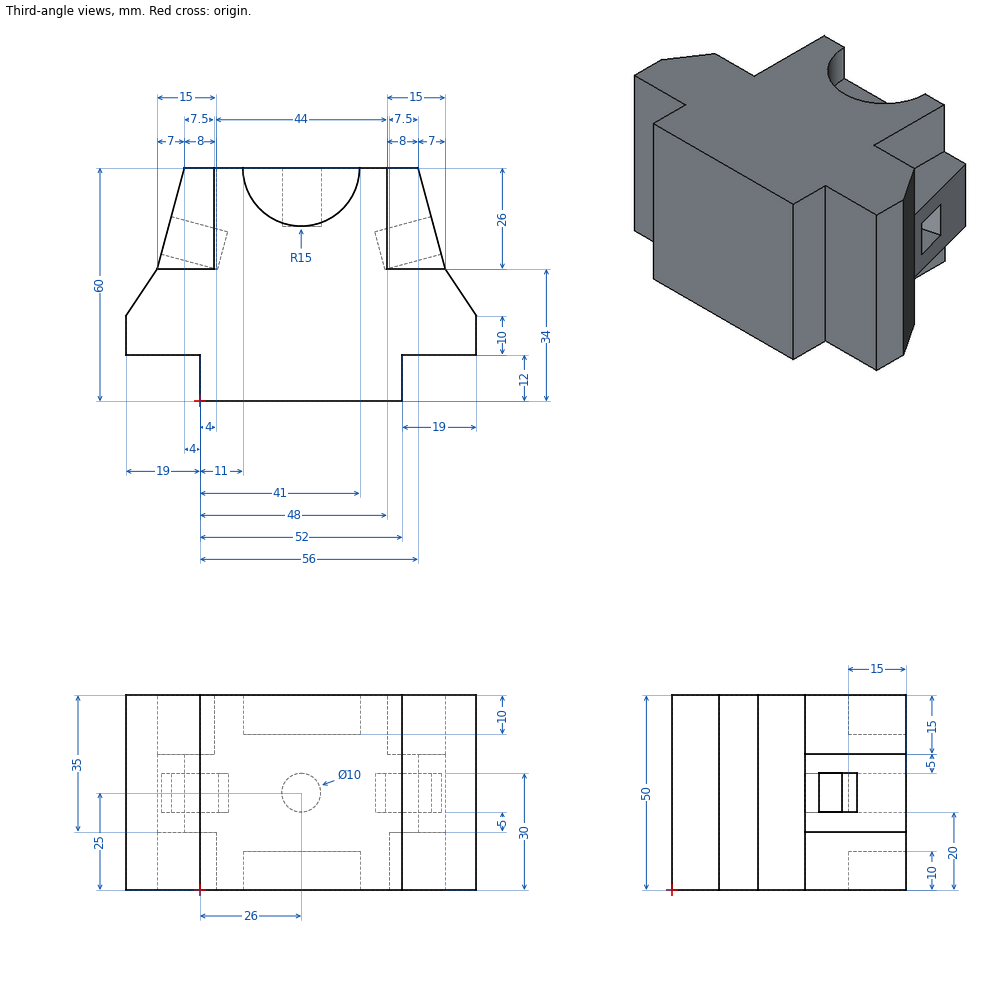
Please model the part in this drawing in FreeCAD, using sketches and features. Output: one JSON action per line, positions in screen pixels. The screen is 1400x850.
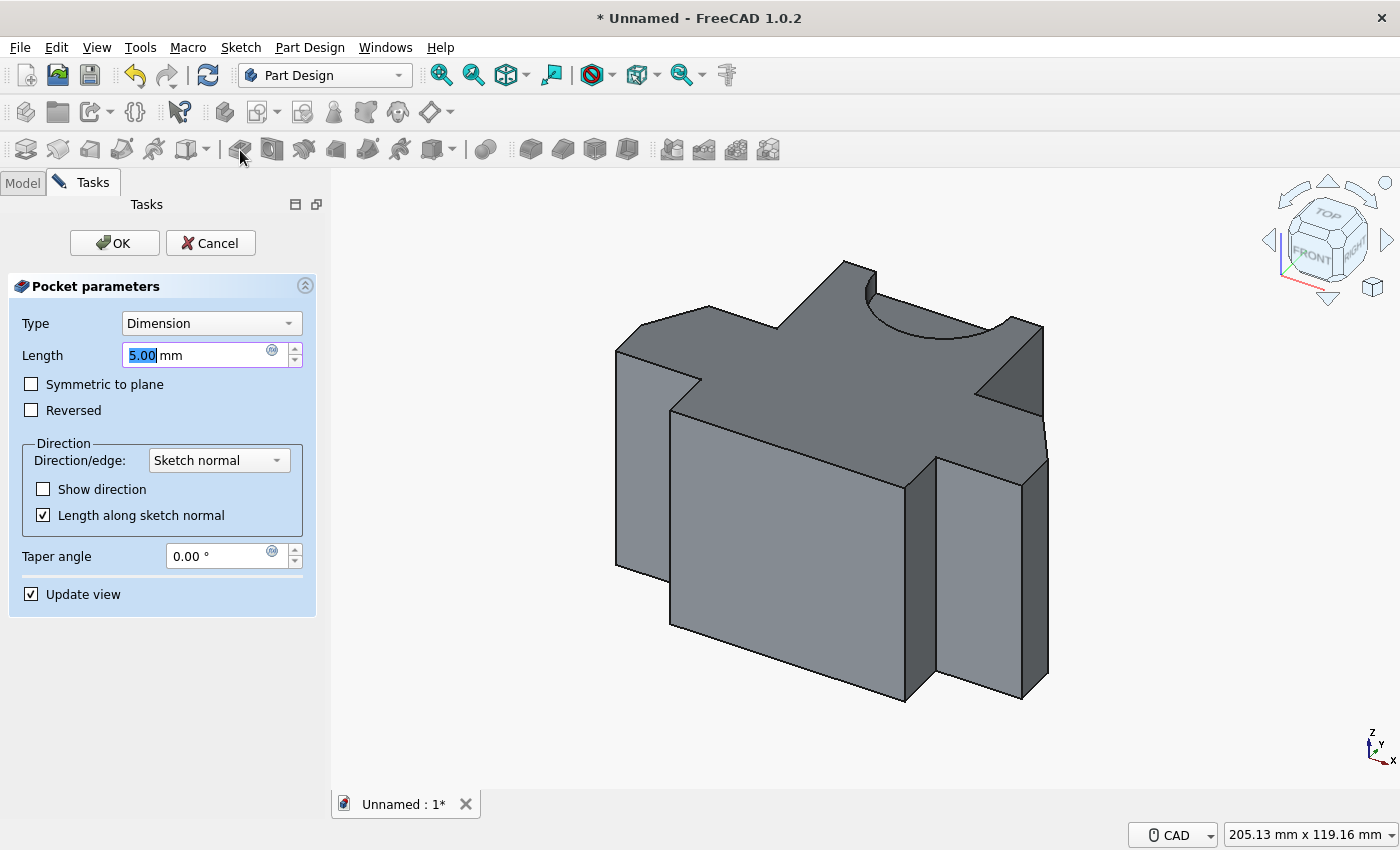
{"action": "type", "text": "10"}
{"action": "key", "text": "Tab"}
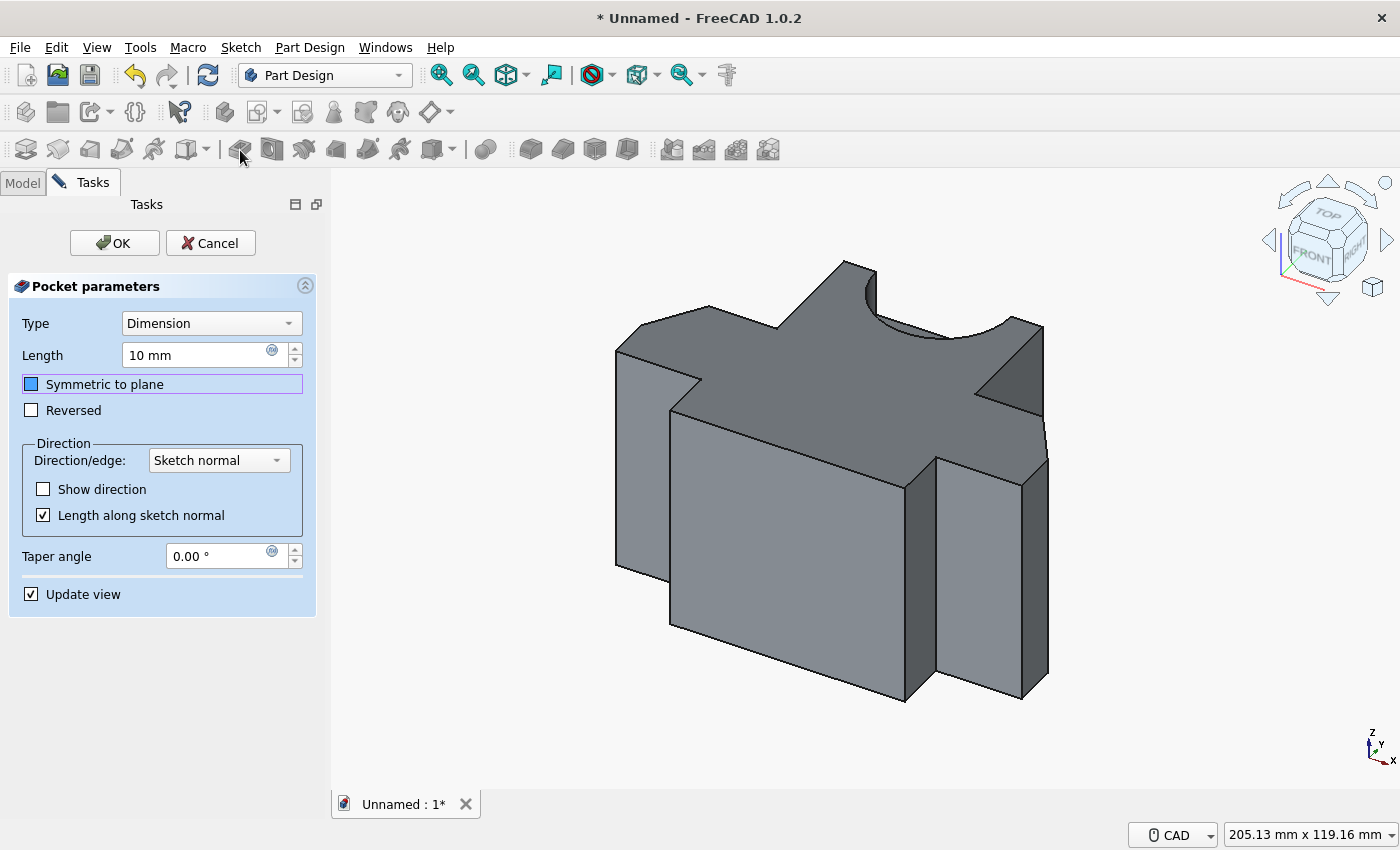
{"action": "left_click", "coordinate": [115, 243]}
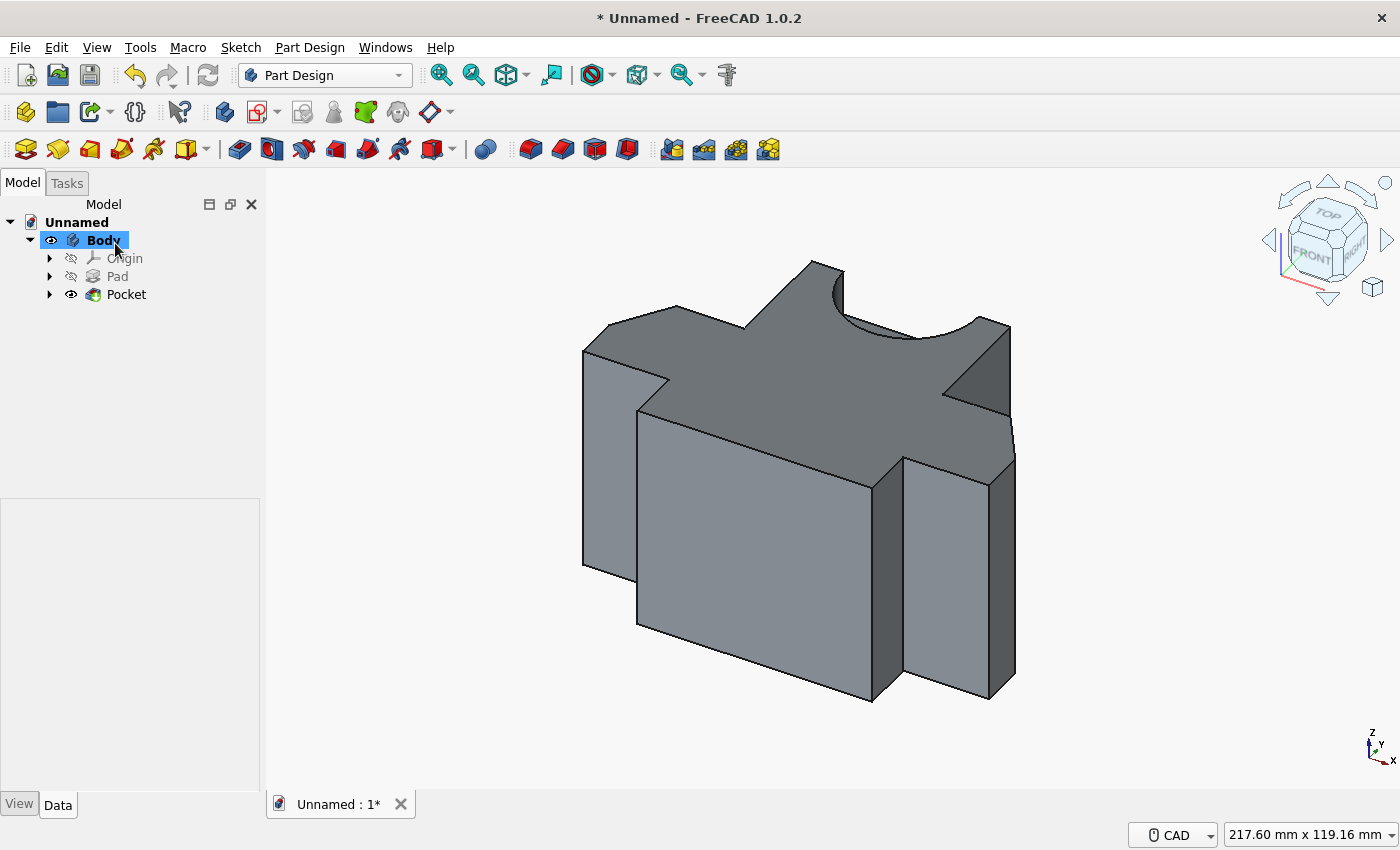
{"action": "left_click", "coordinate": [50, 258]}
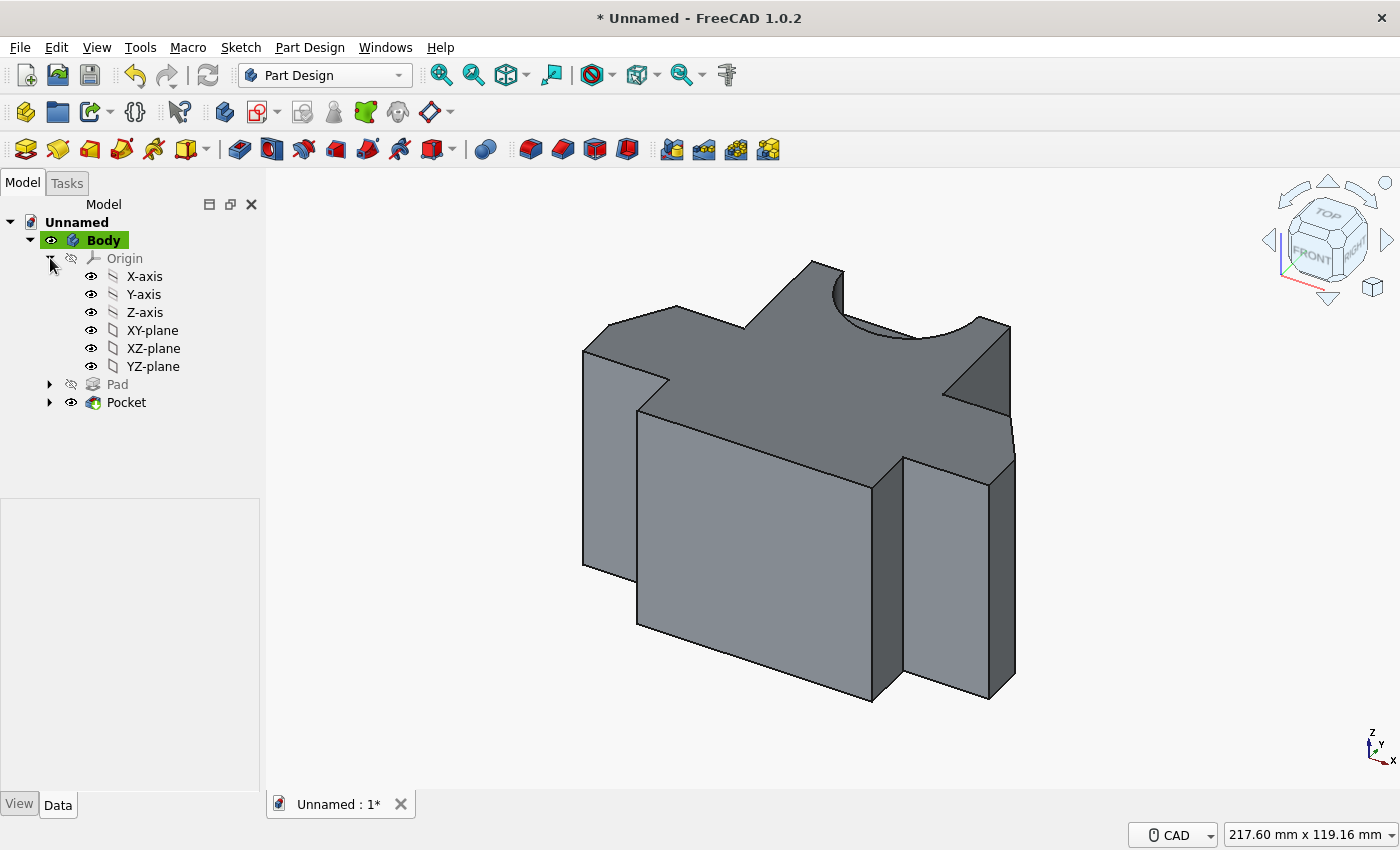
{"action": "left_click", "coordinate": [136, 330]}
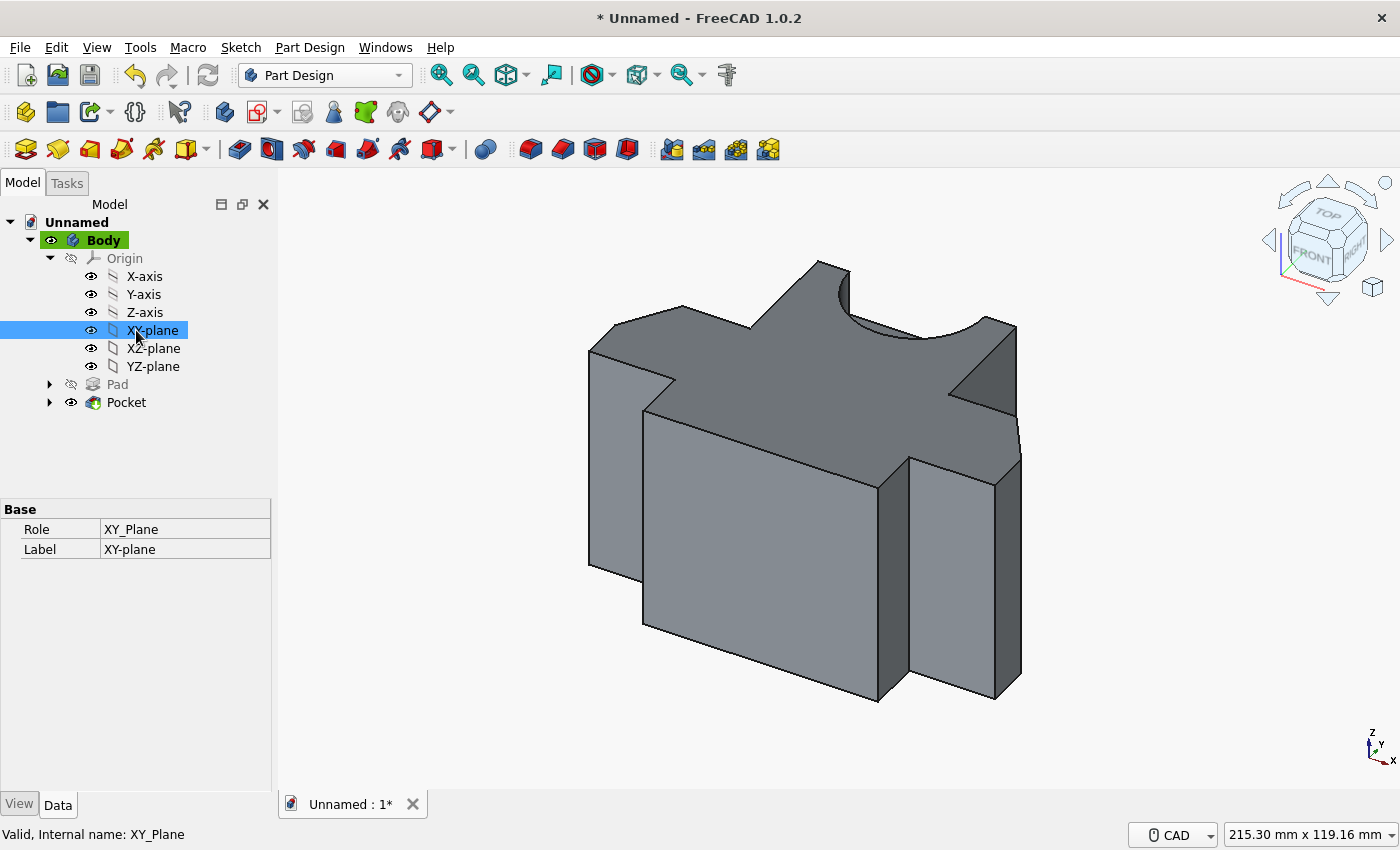
{"action": "left_click", "coordinate": [430, 112]}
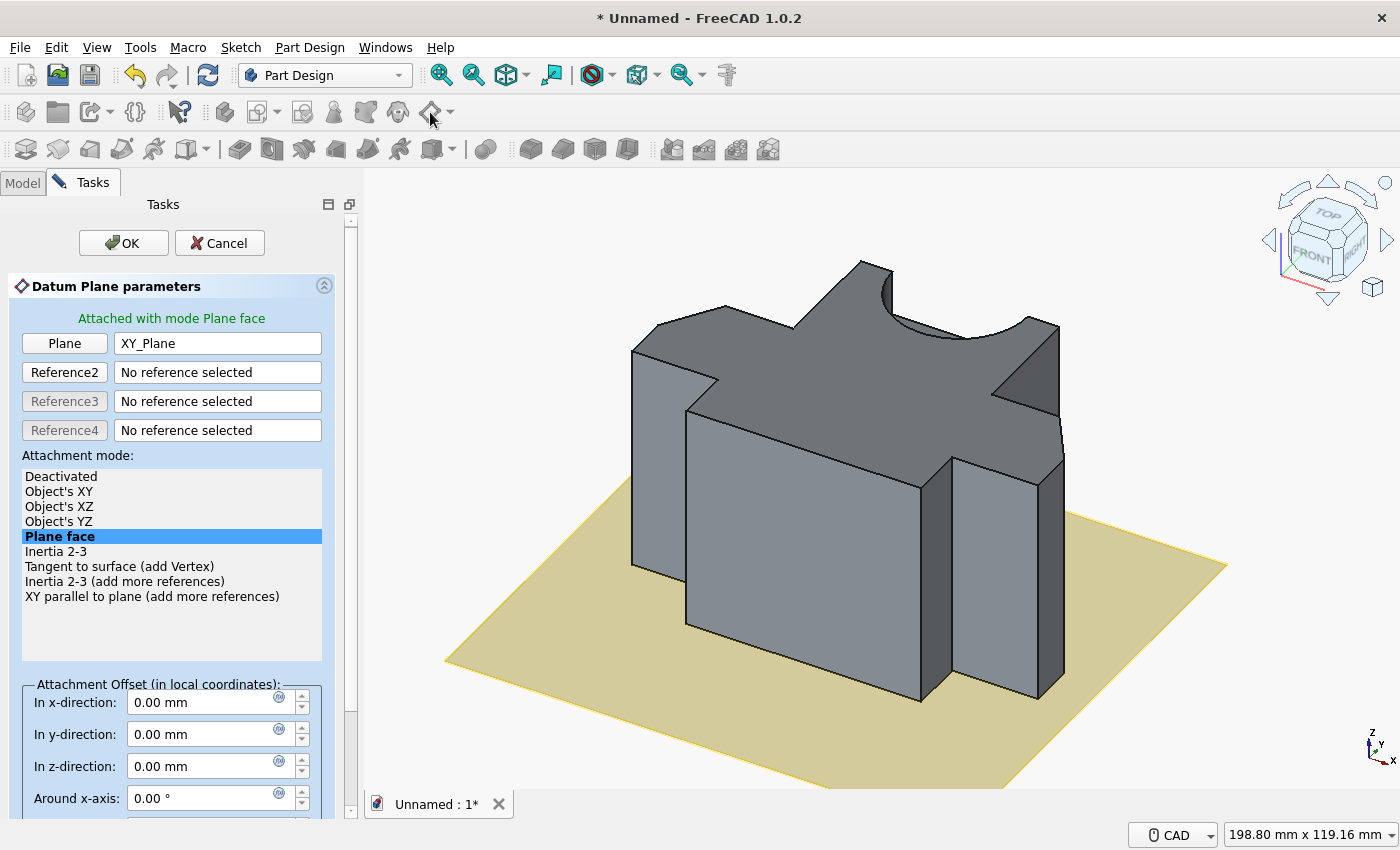
{"action": "triple_click", "coordinate": [210, 766]}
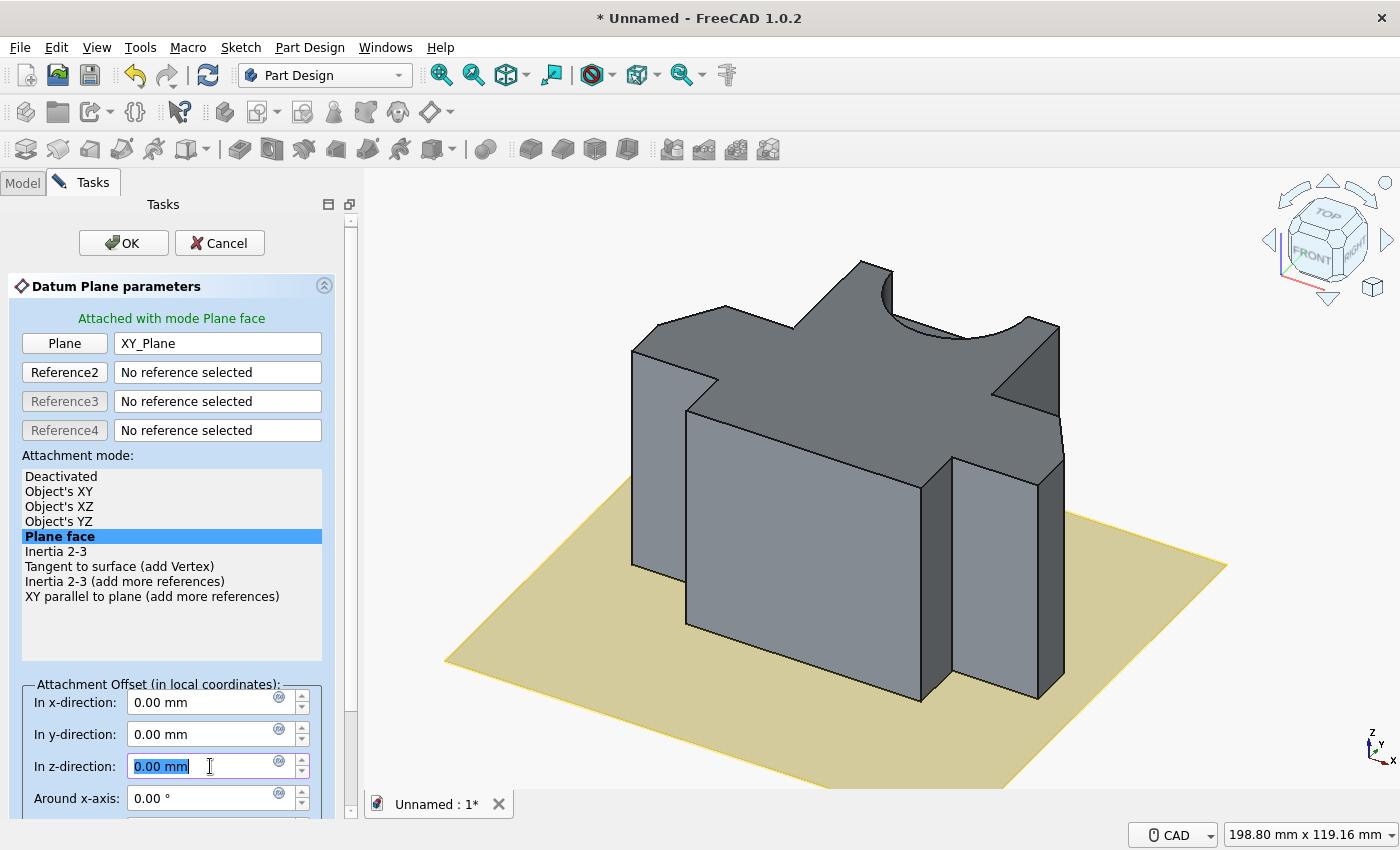
{"action": "type", "text": "10"}
{"action": "key", "text": "Tab"}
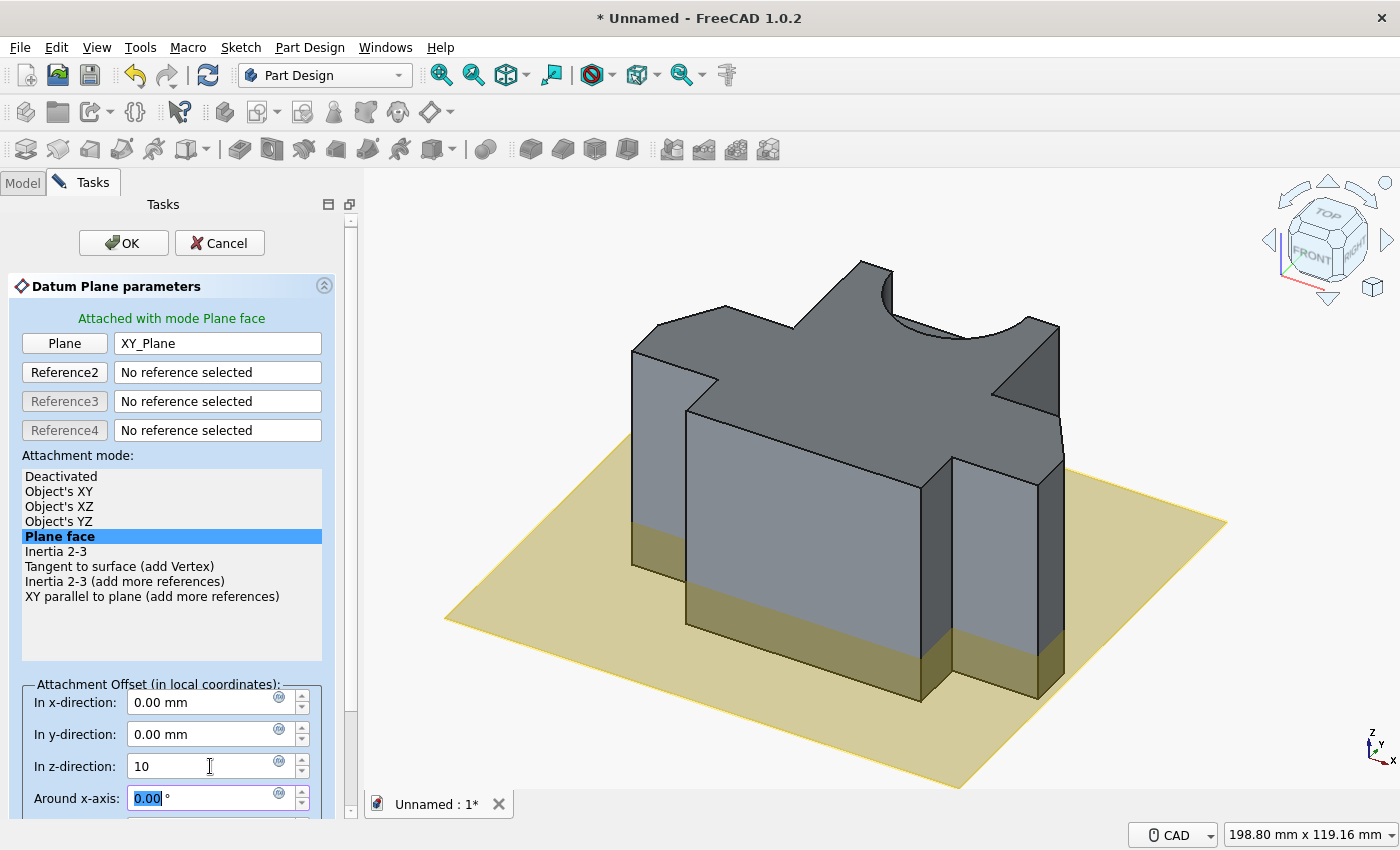
{"action": "left_click", "coordinate": [124, 243]}